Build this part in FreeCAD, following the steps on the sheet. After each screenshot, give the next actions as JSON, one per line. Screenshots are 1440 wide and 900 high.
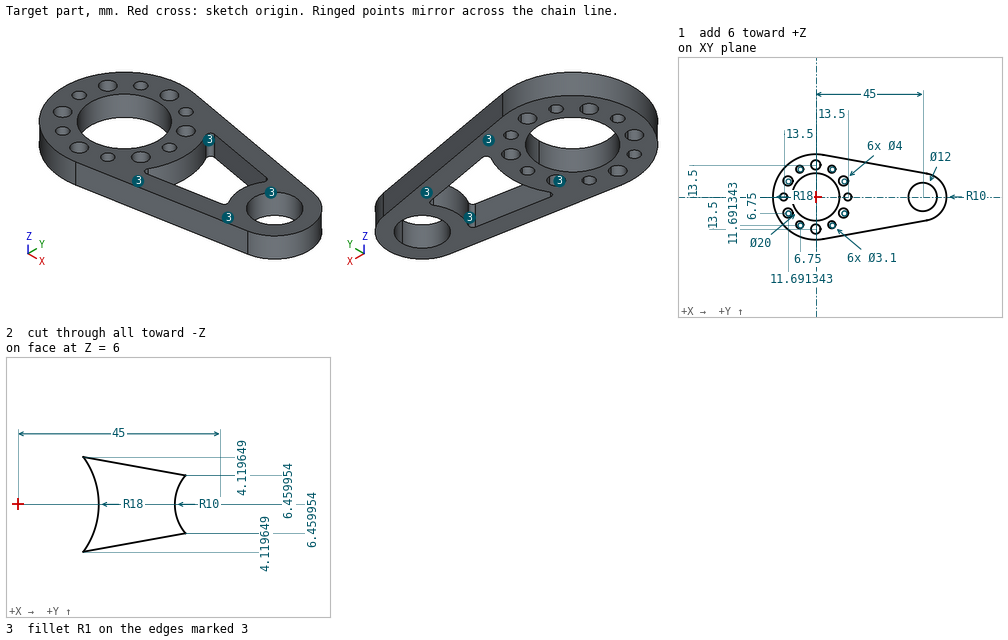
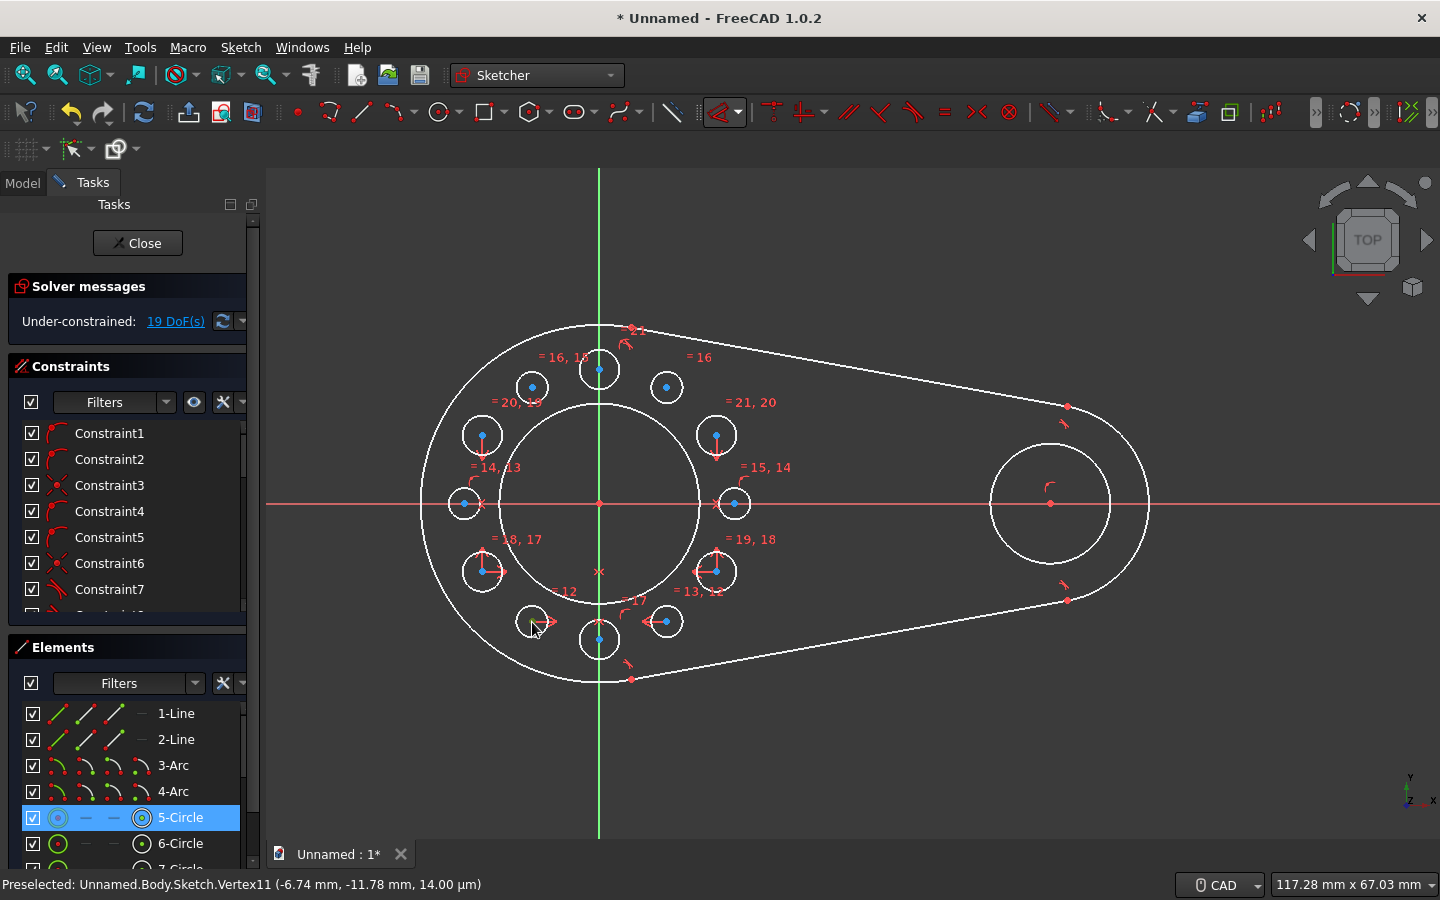
{"action": "left_click", "coordinate": [532, 388]}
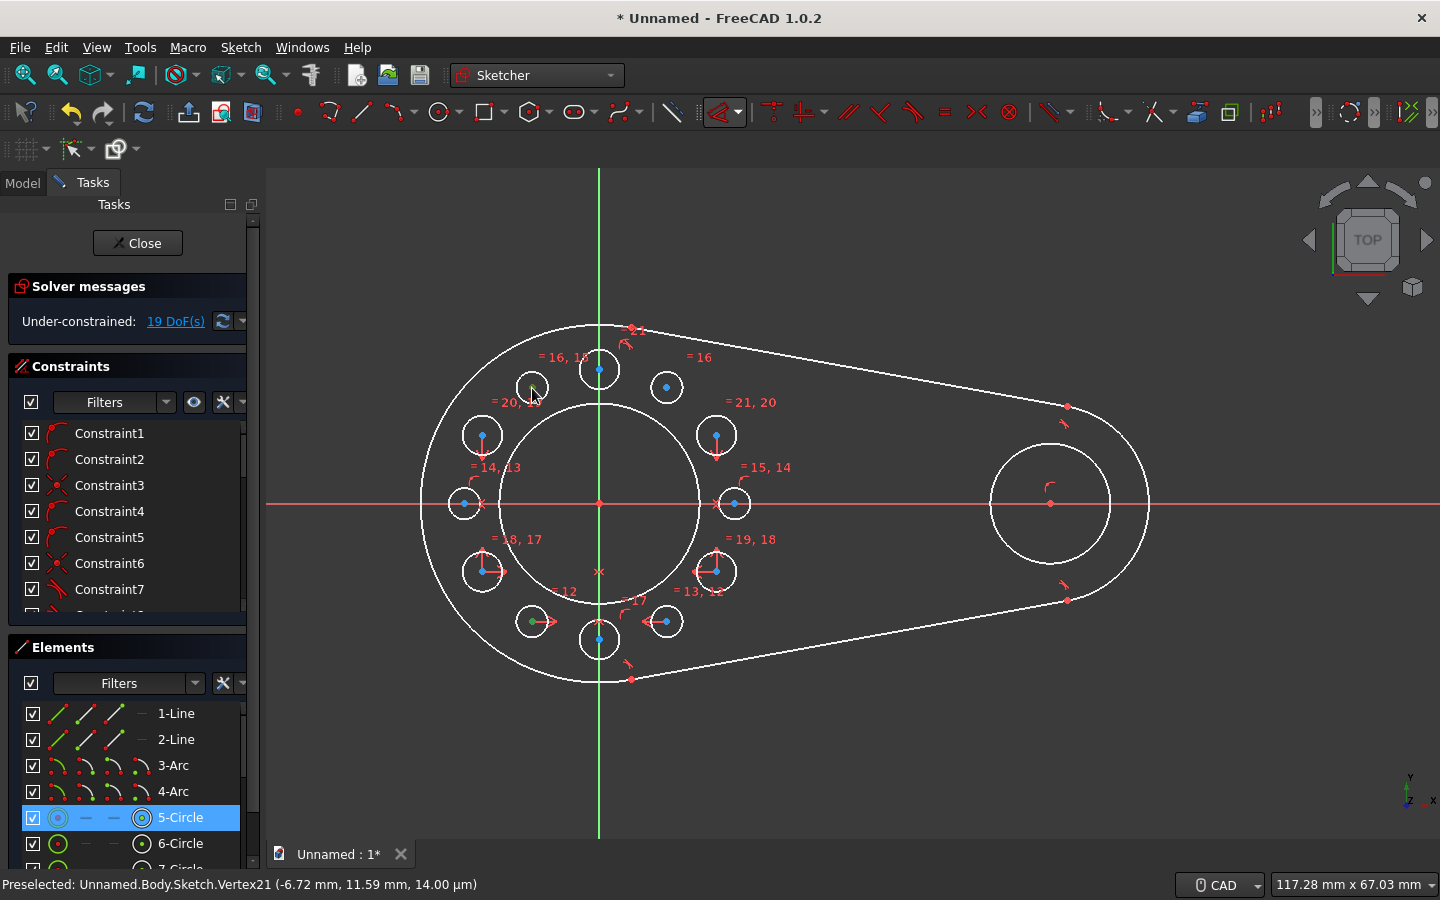
{"action": "left_click", "coordinate": [364, 504]}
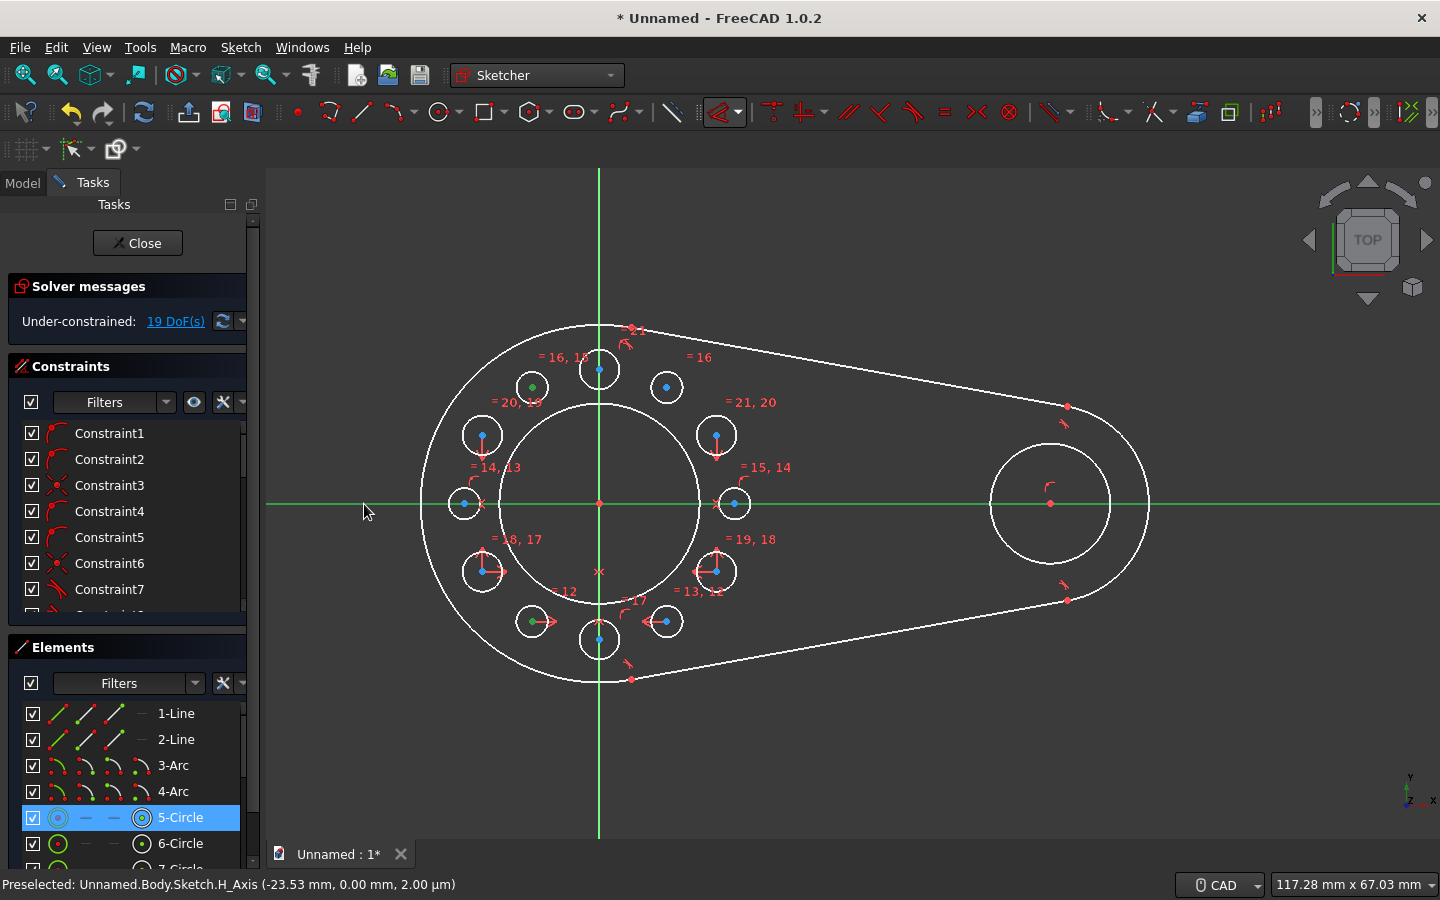
{"action": "left_click", "coordinate": [978, 112]}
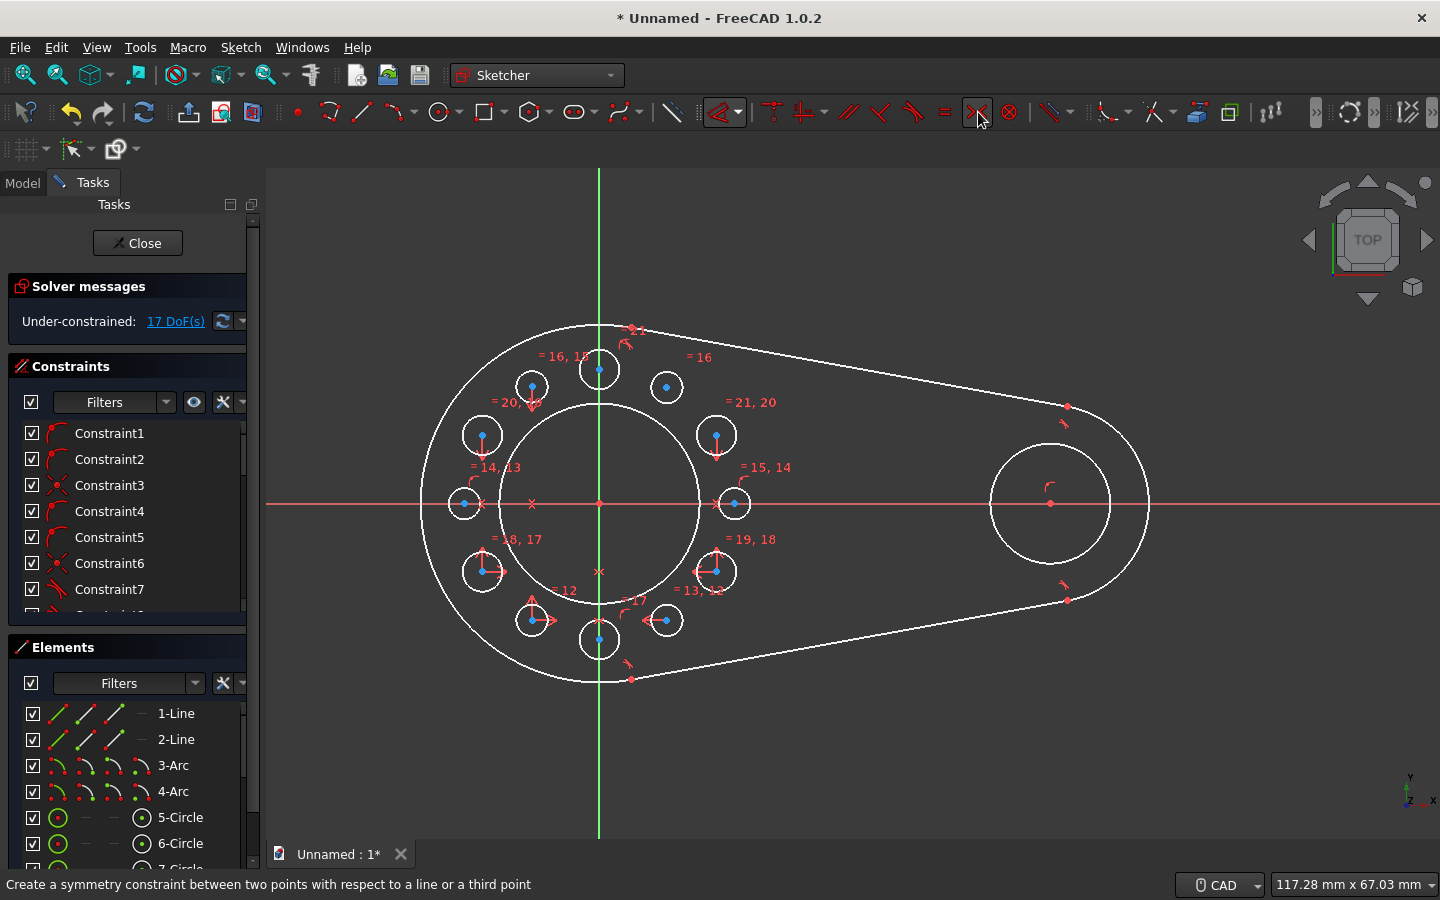
{"action": "left_click", "coordinate": [667, 620]}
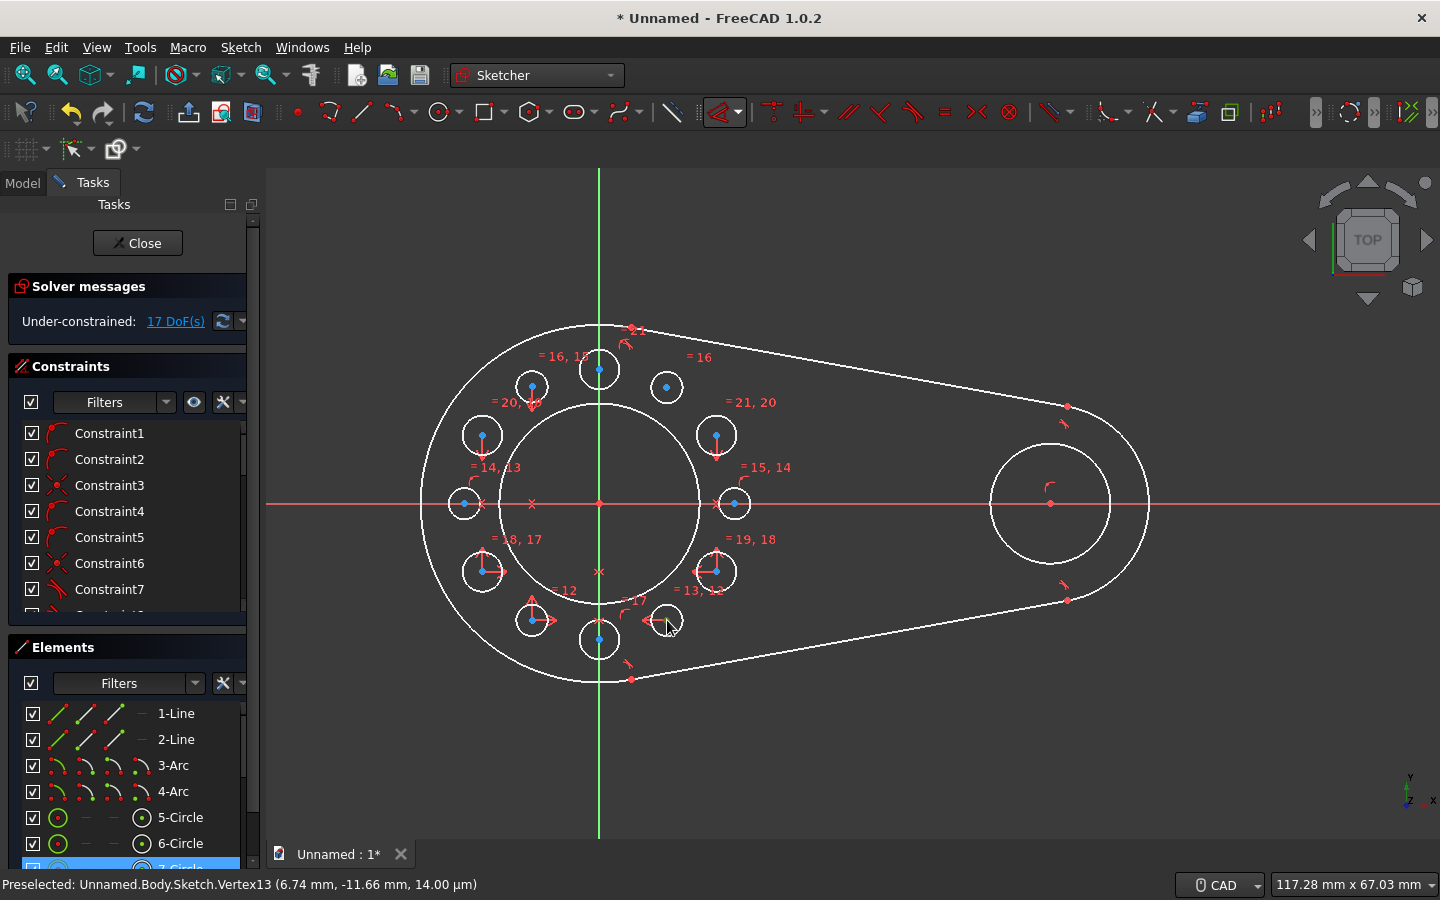
{"action": "left_click", "coordinate": [667, 388]}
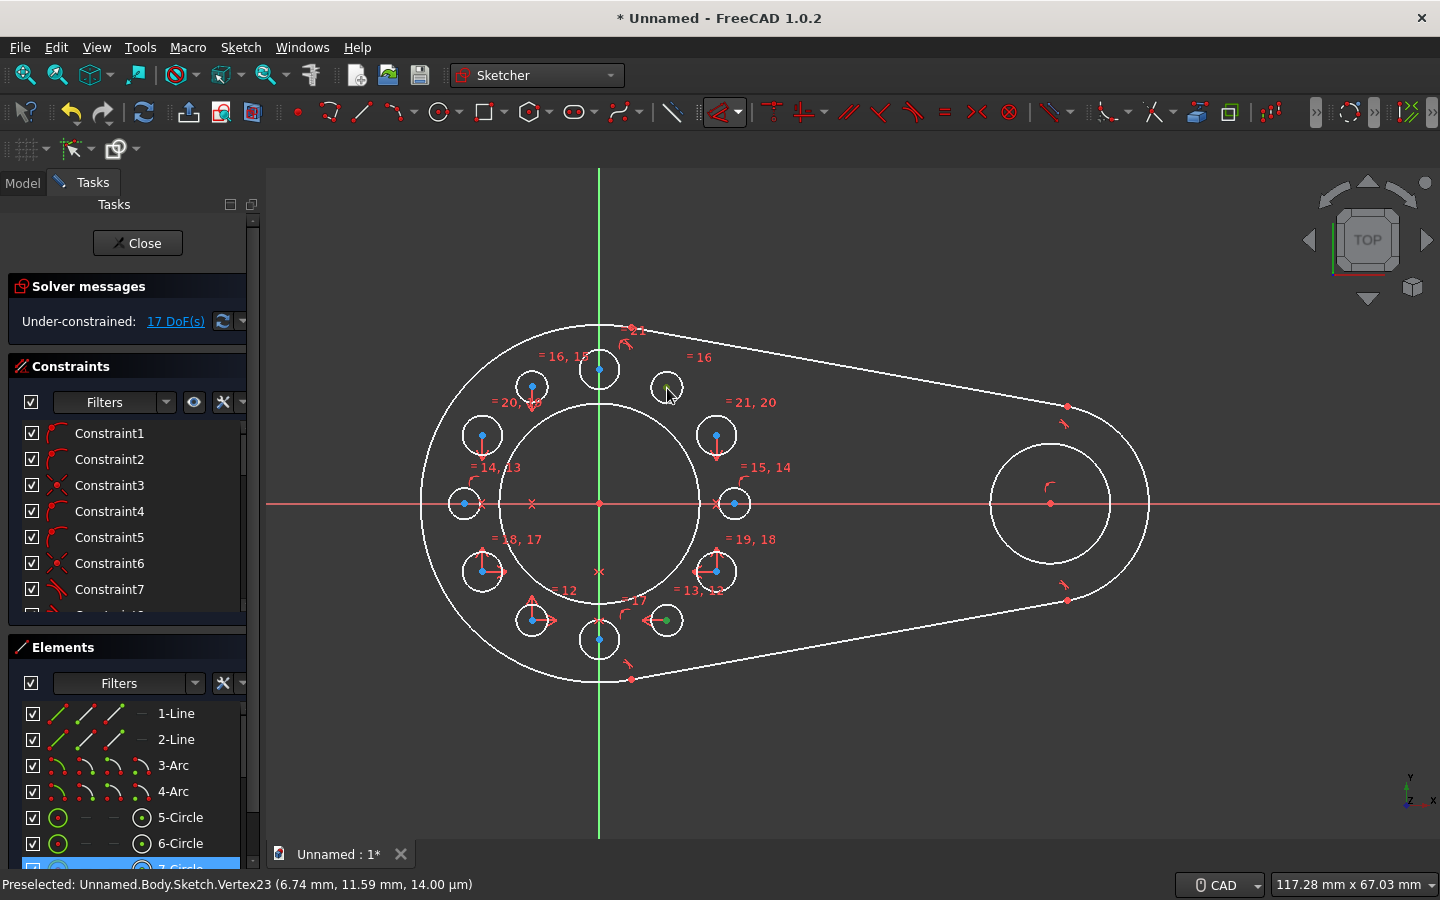
{"action": "left_click", "coordinate": [364, 504]}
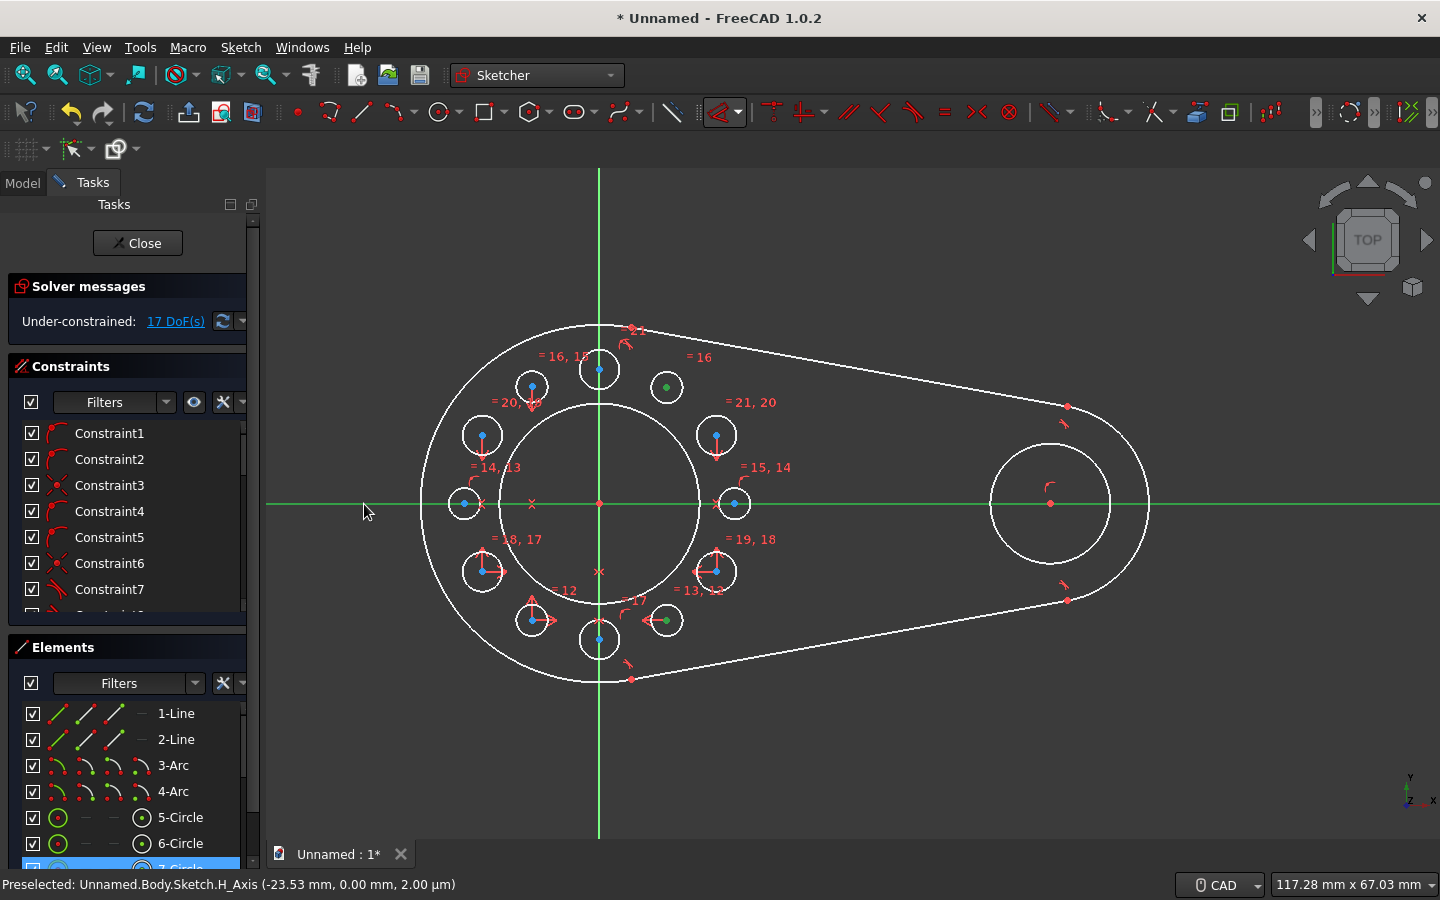
{"action": "key", "text": "s"}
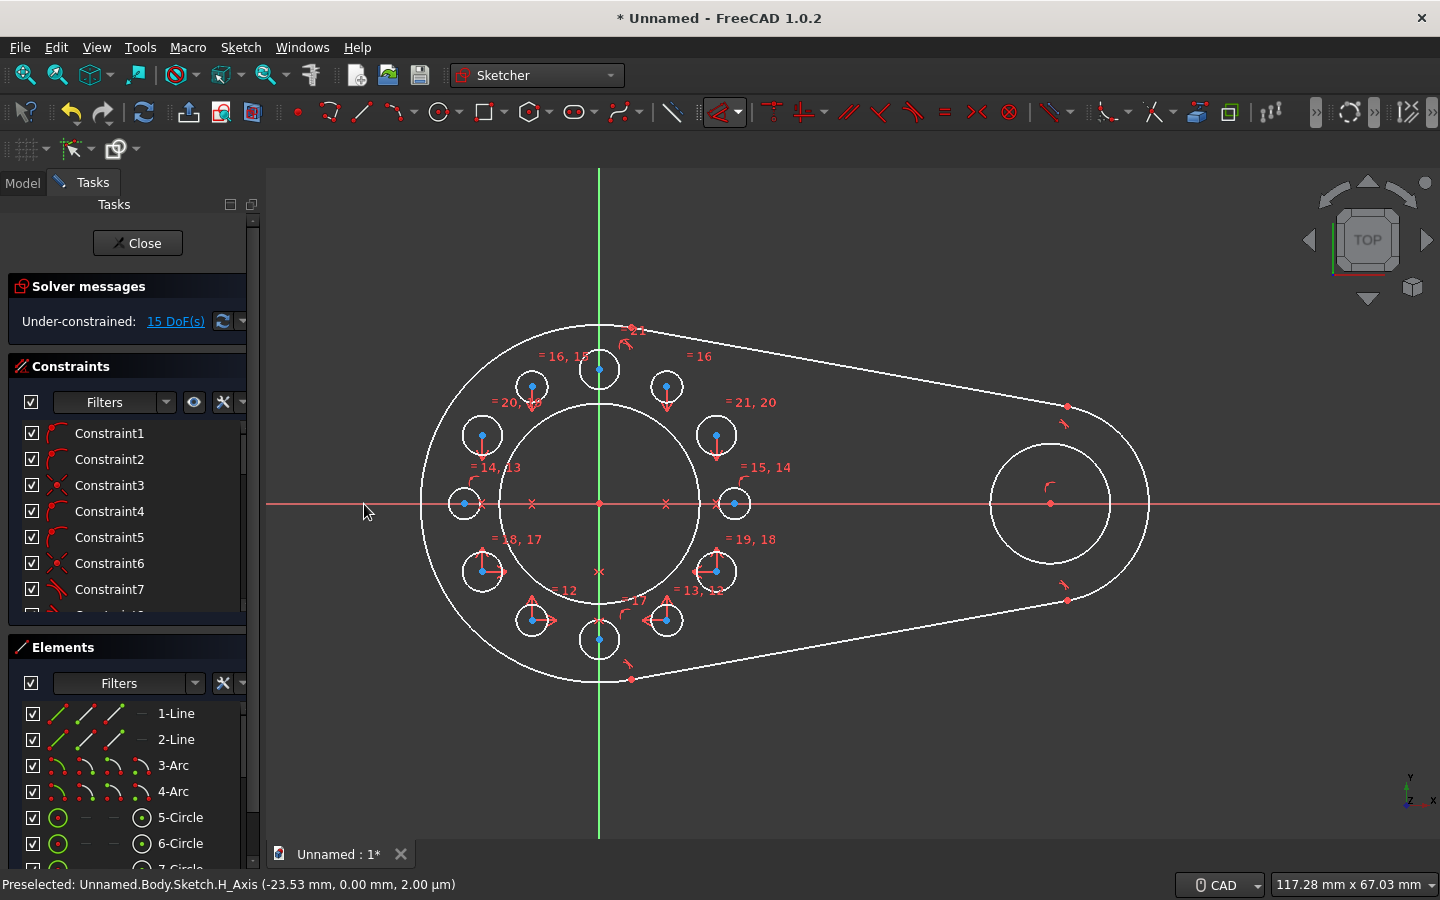
{"action": "key", "text": "d"}